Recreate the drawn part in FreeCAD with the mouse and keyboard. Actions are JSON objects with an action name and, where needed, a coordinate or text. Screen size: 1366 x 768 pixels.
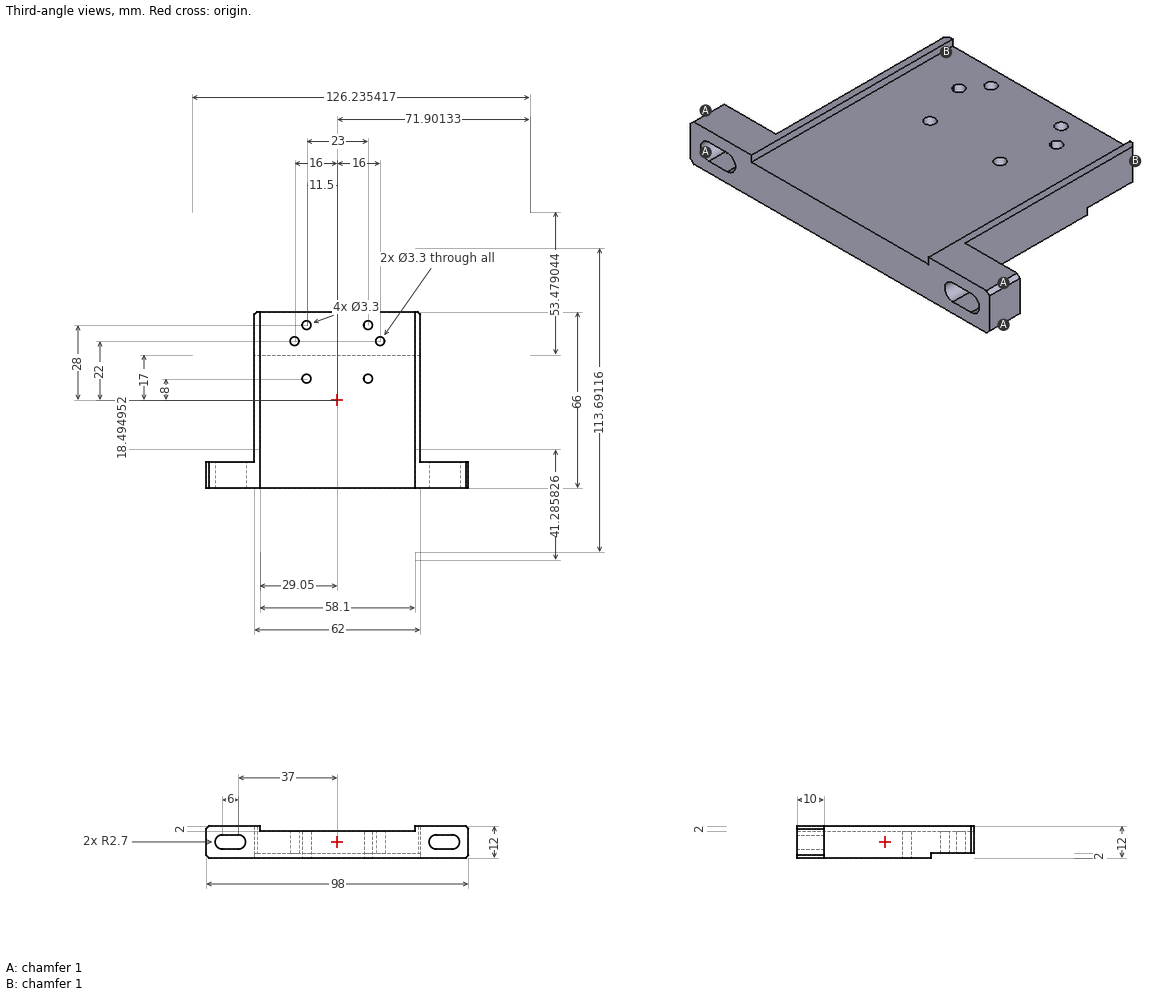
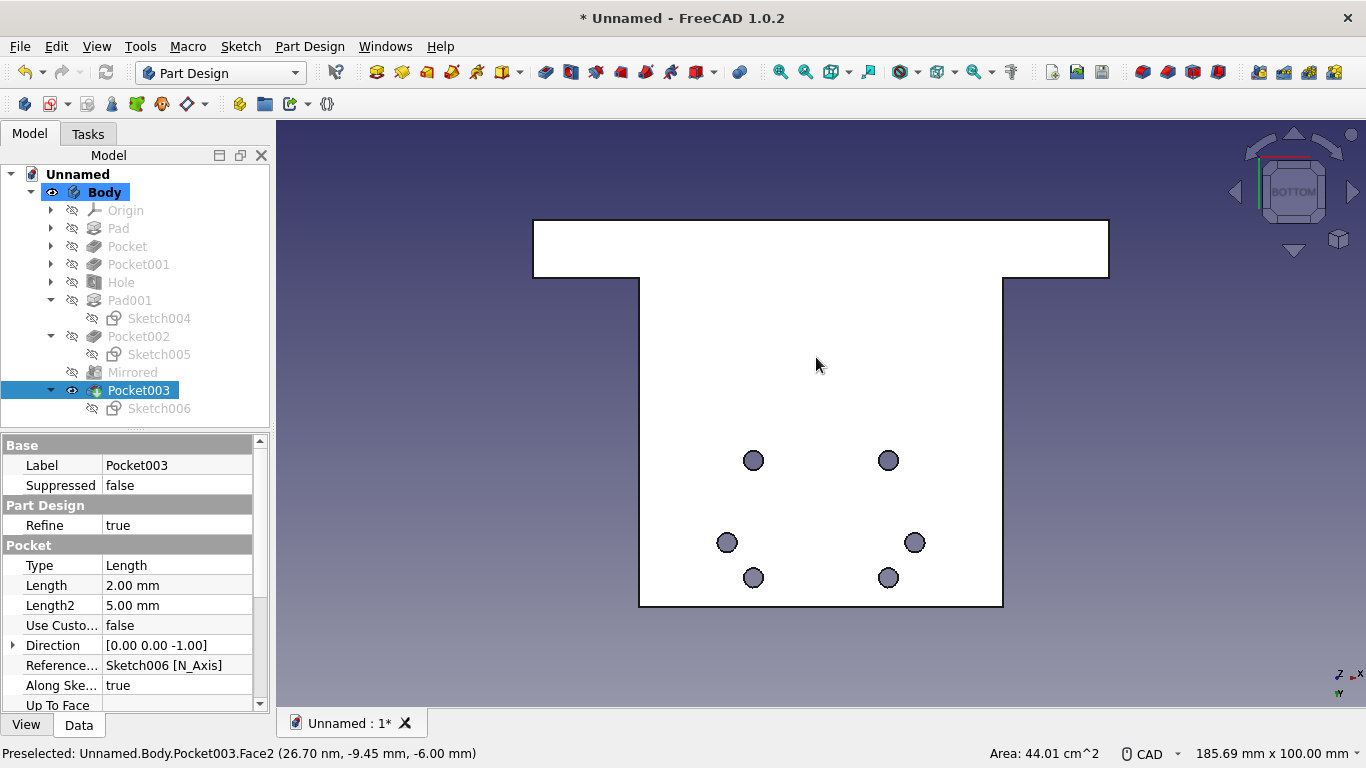
{"action": "left_click", "coordinate": [50, 104]}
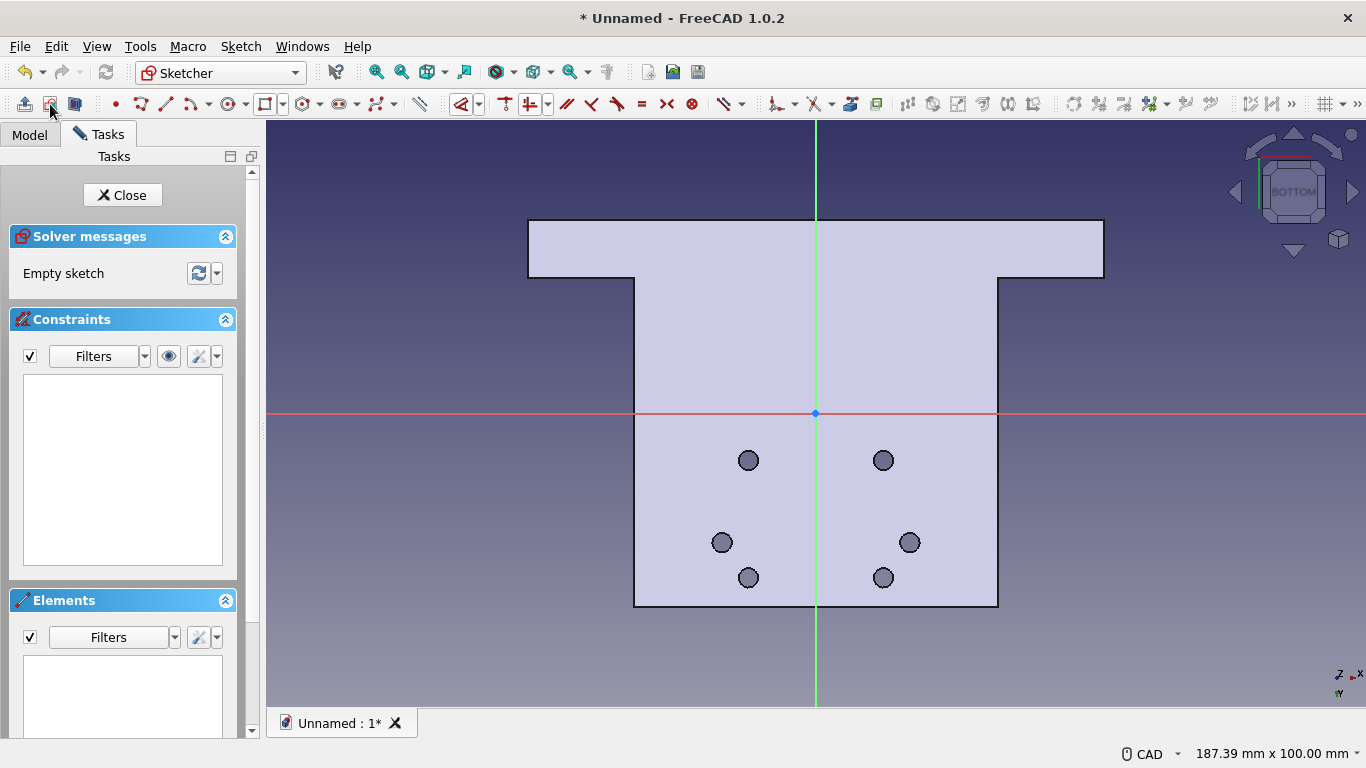
{"action": "scroll", "coordinate": [503, 148], "scroll_direction": "down", "scroll_amount": 2}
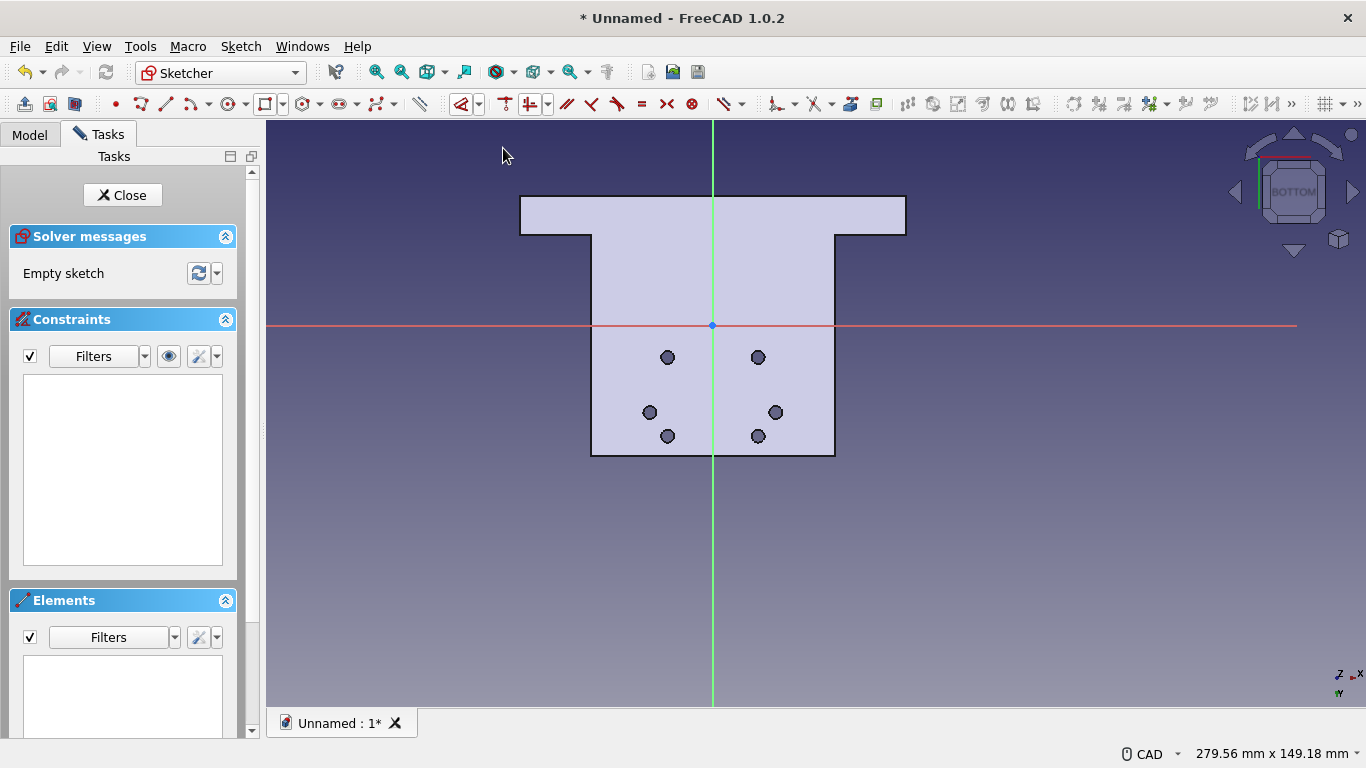
{"action": "left_click", "coordinate": [264, 104]}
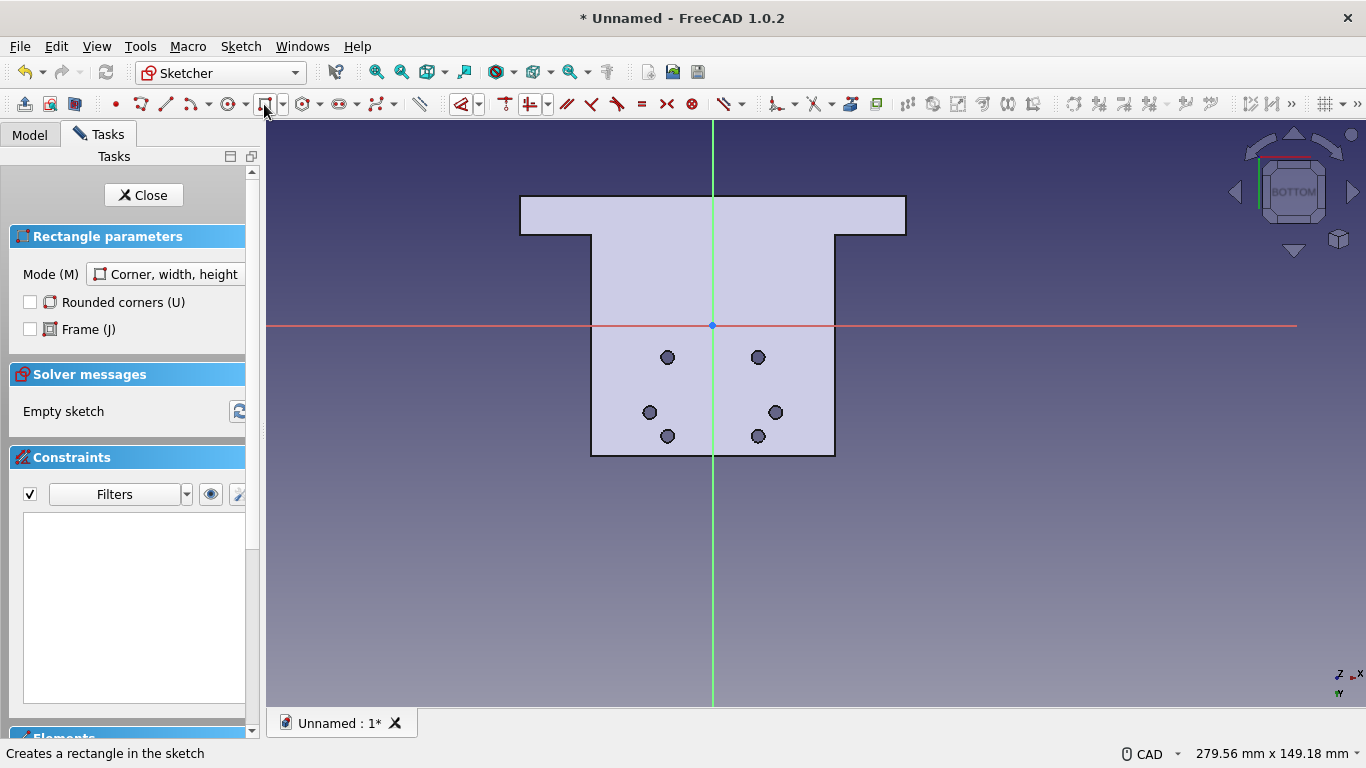
{"action": "left_click", "coordinate": [499, 393]}
{"action": "mouse_move", "coordinate": [996, 603]}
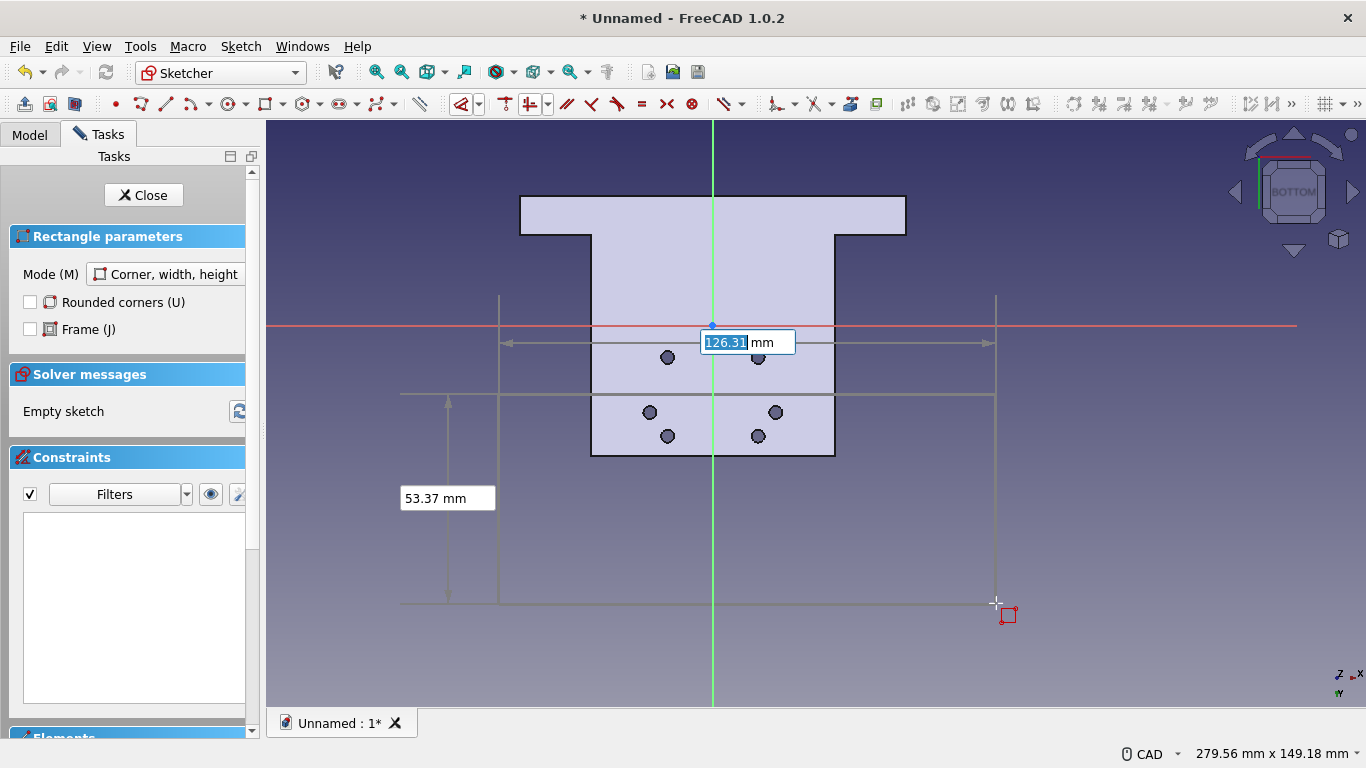
{"action": "type", "text": "126.235417"}
{"action": "key", "text": "Tab"}
{"action": "type", "text": "53.479044"}
{"action": "key", "text": "Return"}
{"action": "key", "text": "Escape"}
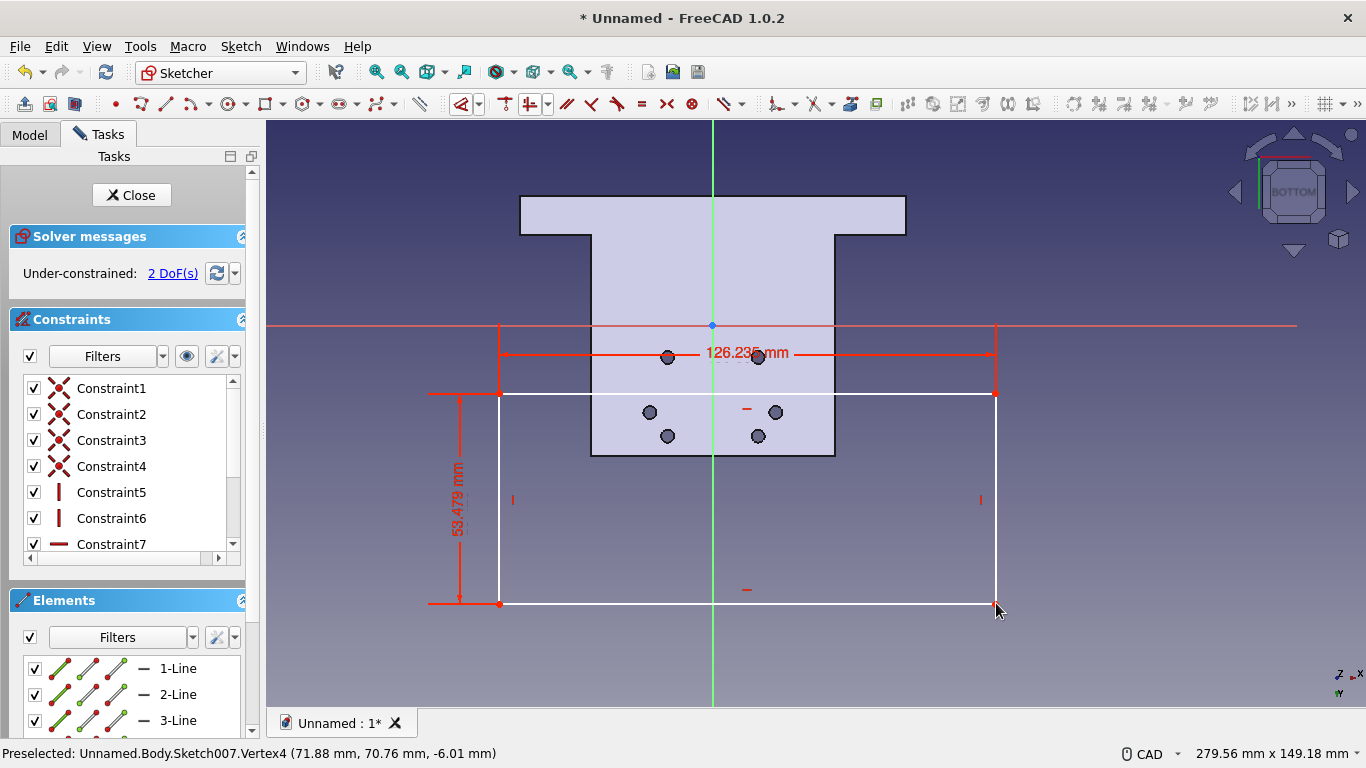
{"action": "left_click", "coordinate": [499, 394]}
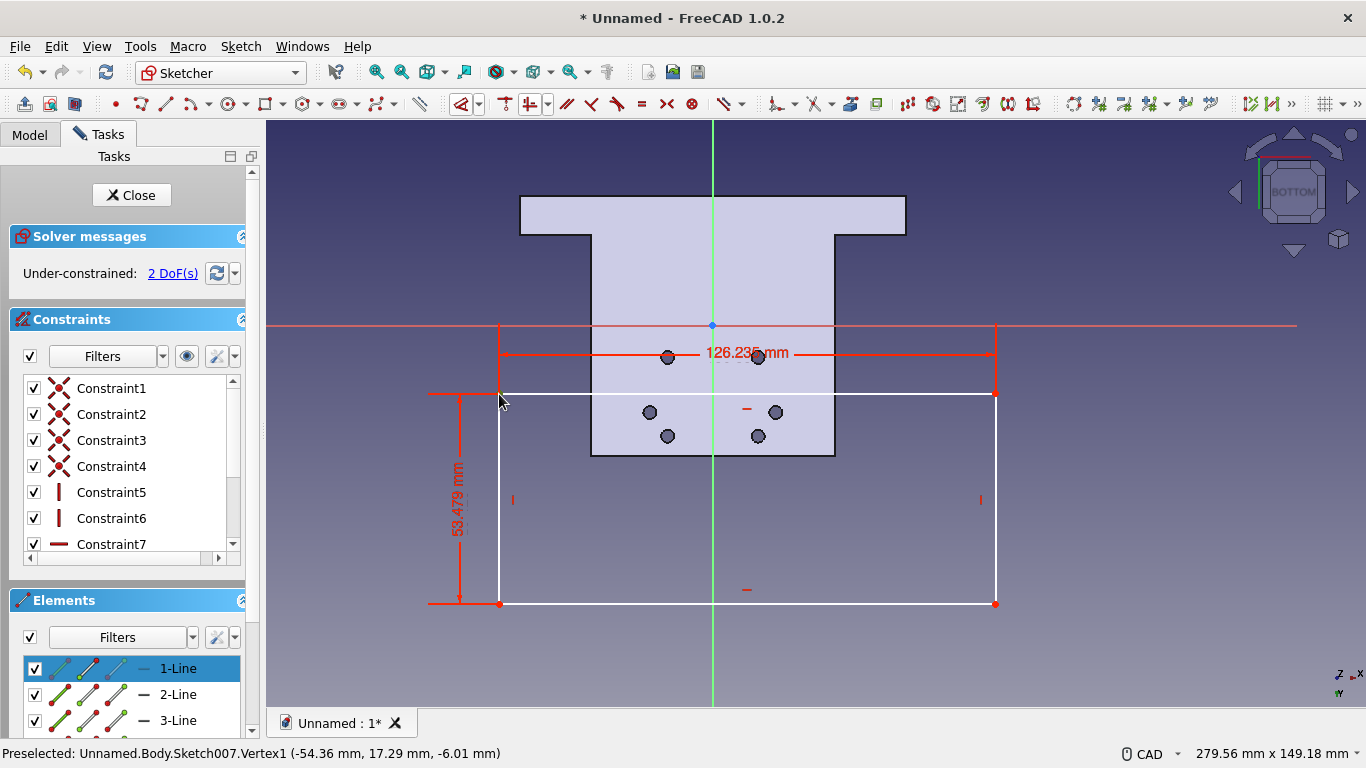
{"action": "left_click", "coordinate": [478, 104]}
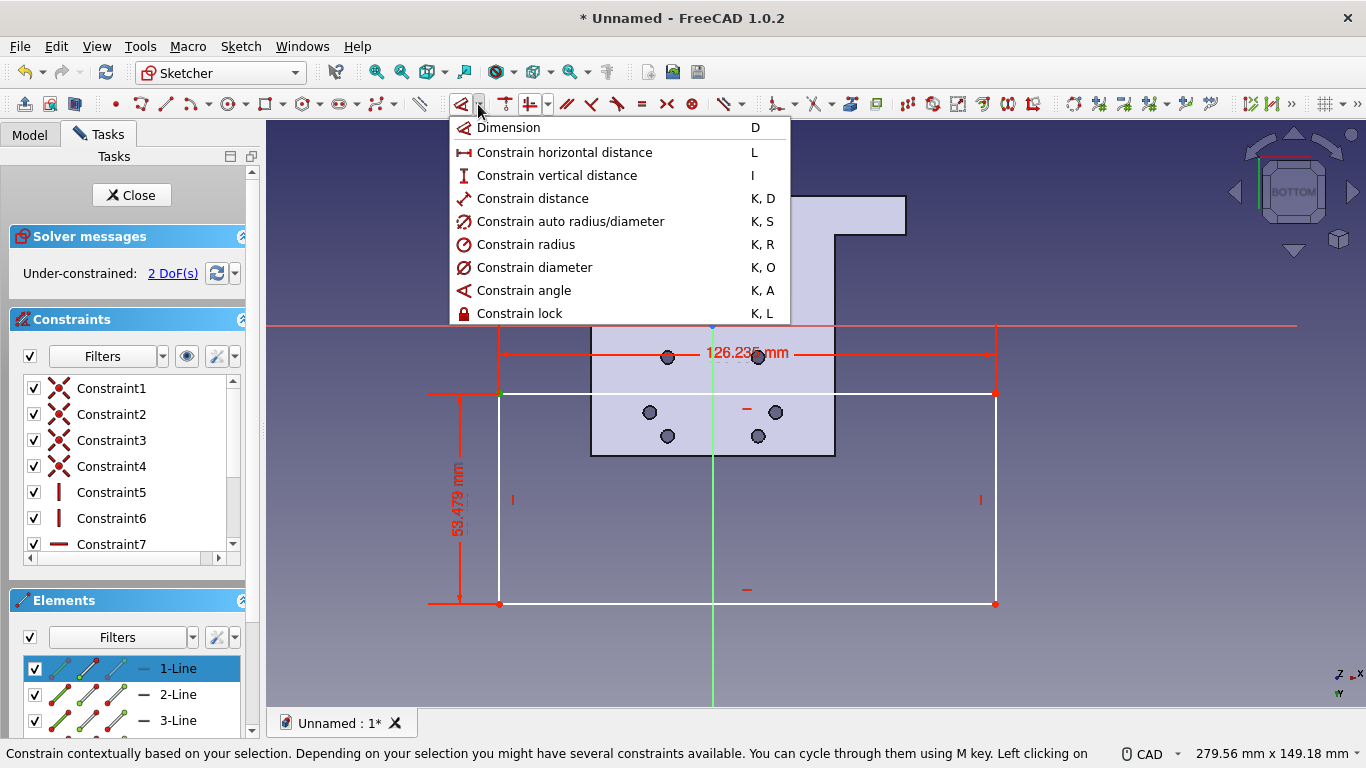
{"action": "left_click", "coordinate": [620, 176]}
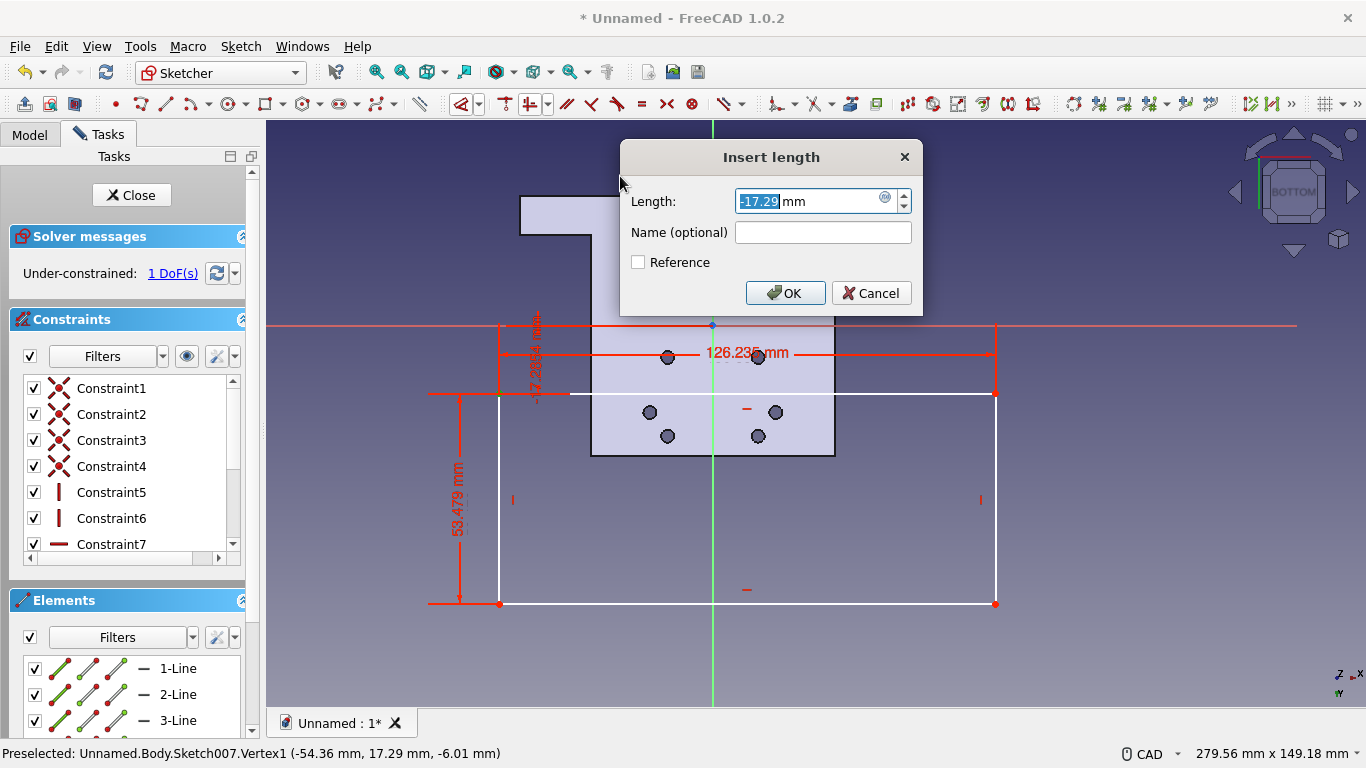
{"action": "type", "text": "-17"}
{"action": "key", "text": "Return"}